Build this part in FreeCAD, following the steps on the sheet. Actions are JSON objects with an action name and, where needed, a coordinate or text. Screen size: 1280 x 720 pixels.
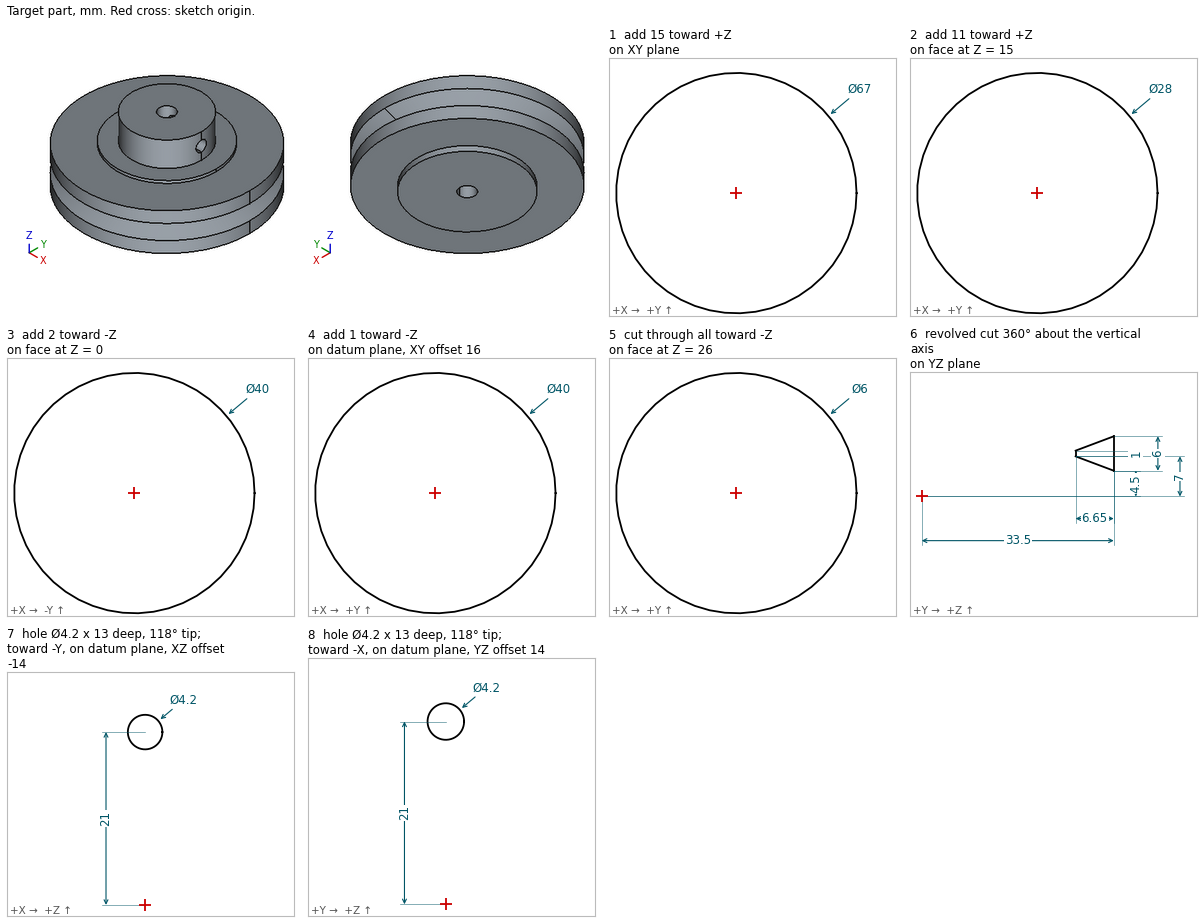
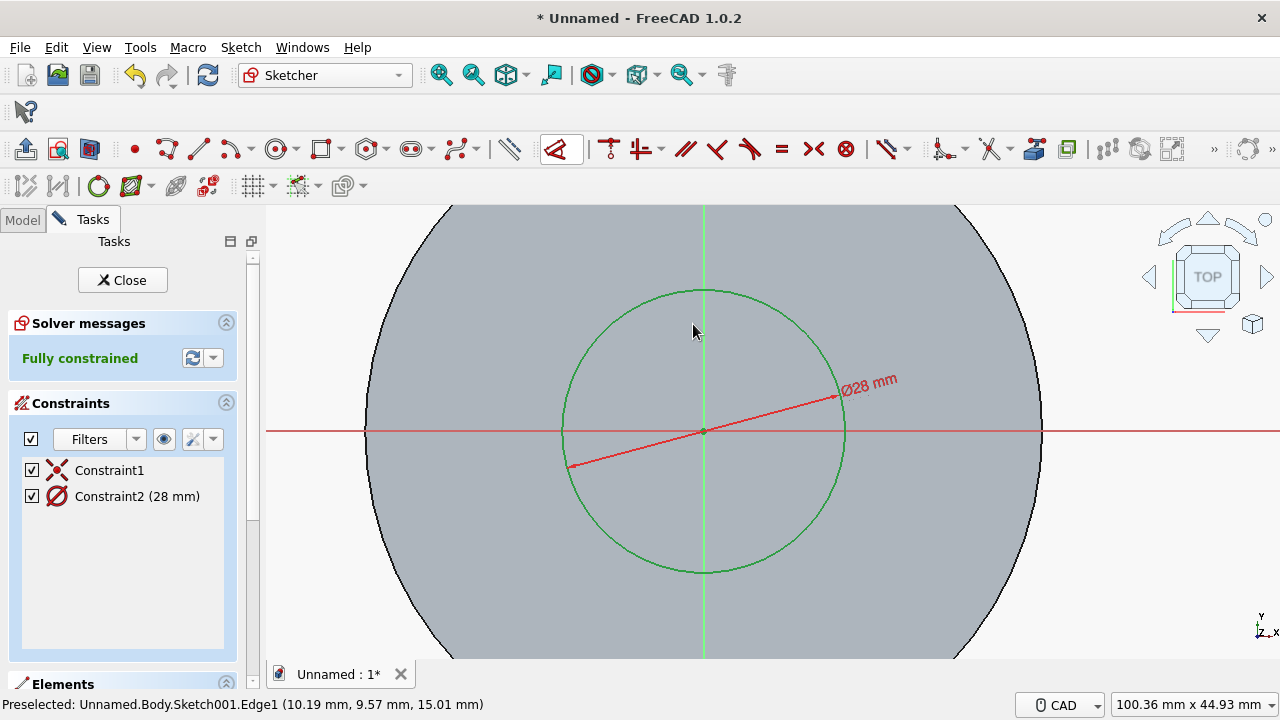
{"action": "left_click", "coordinate": [123, 280]}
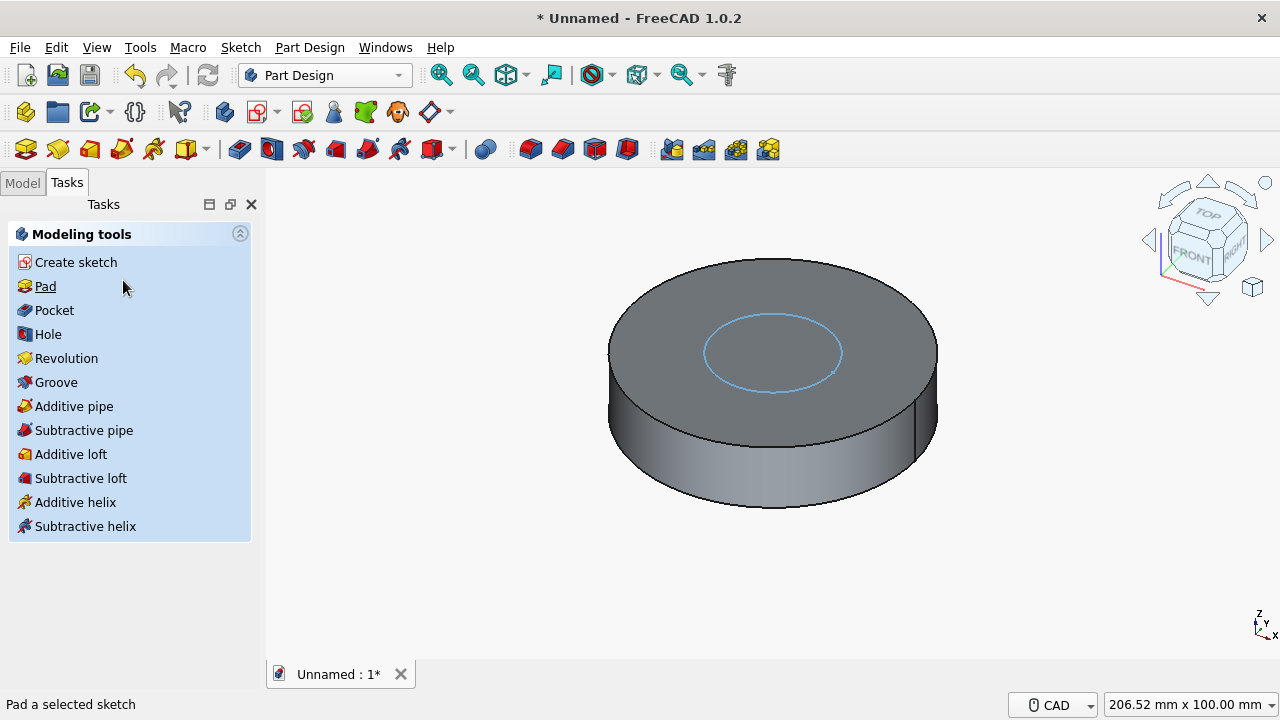
{"action": "left_click", "coordinate": [26, 150]}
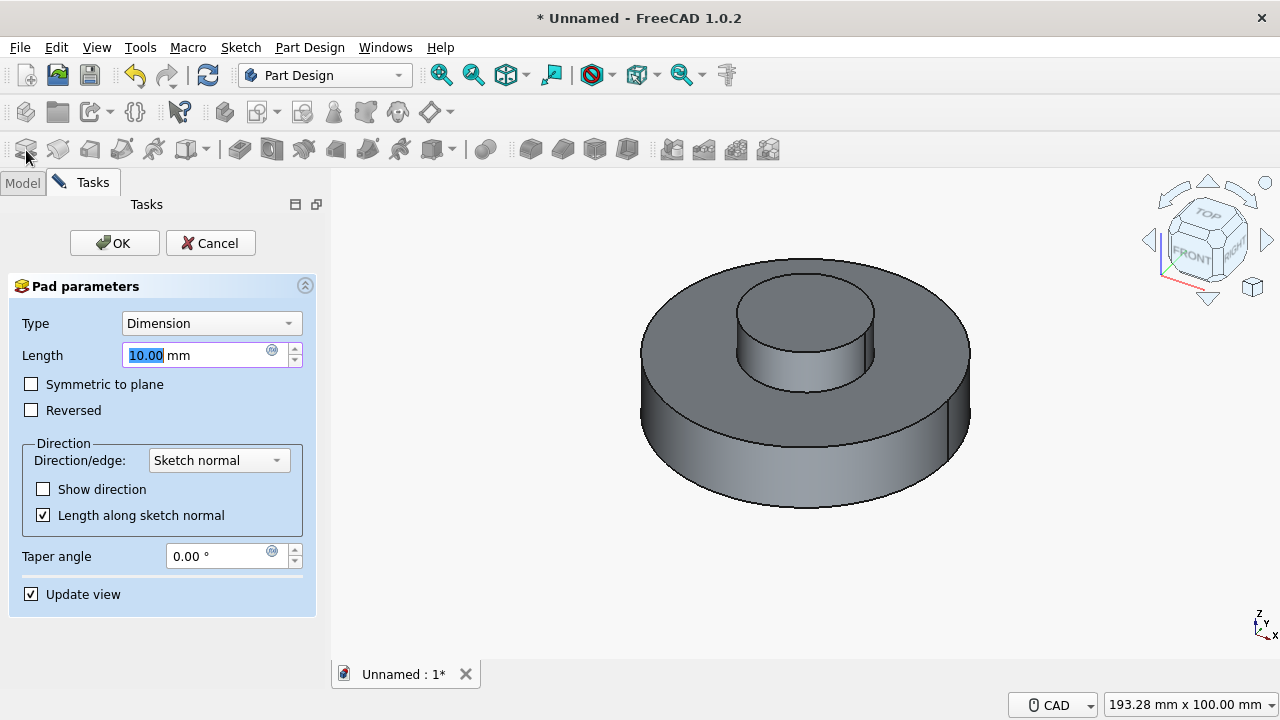
{"action": "type", "text": "11"}
{"action": "key", "text": "Tab"}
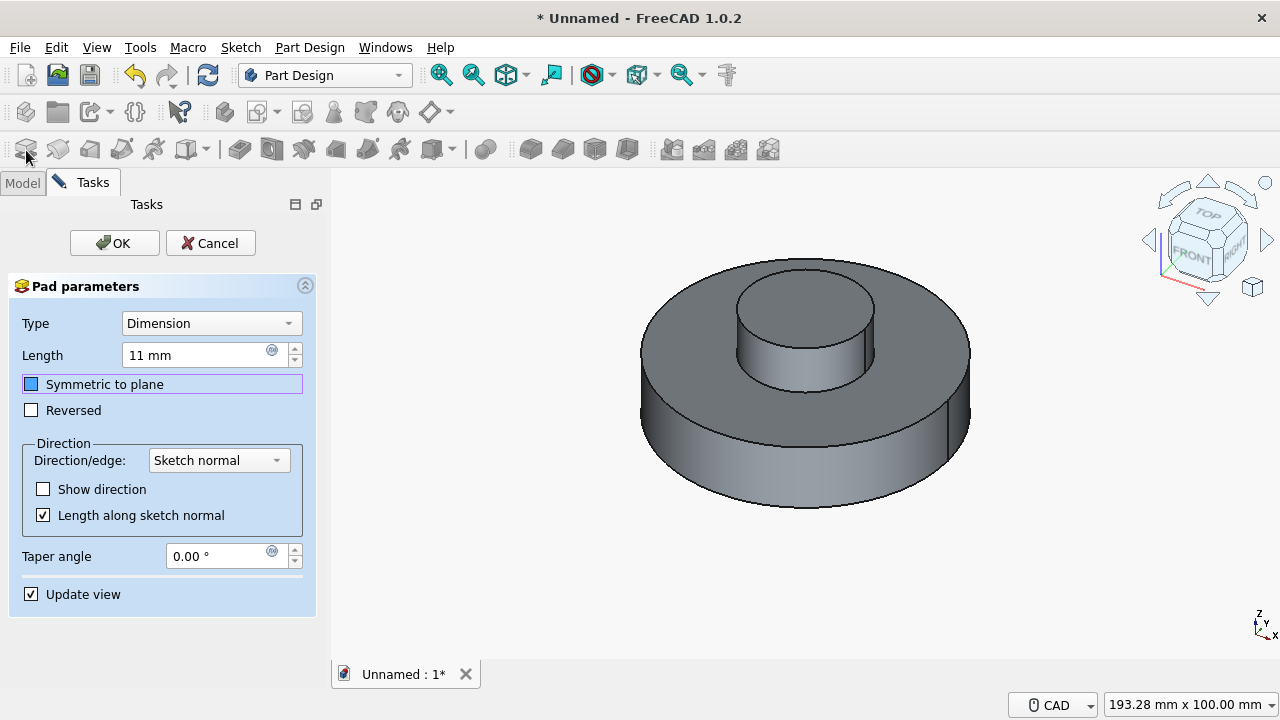
{"action": "left_click", "coordinate": [115, 243]}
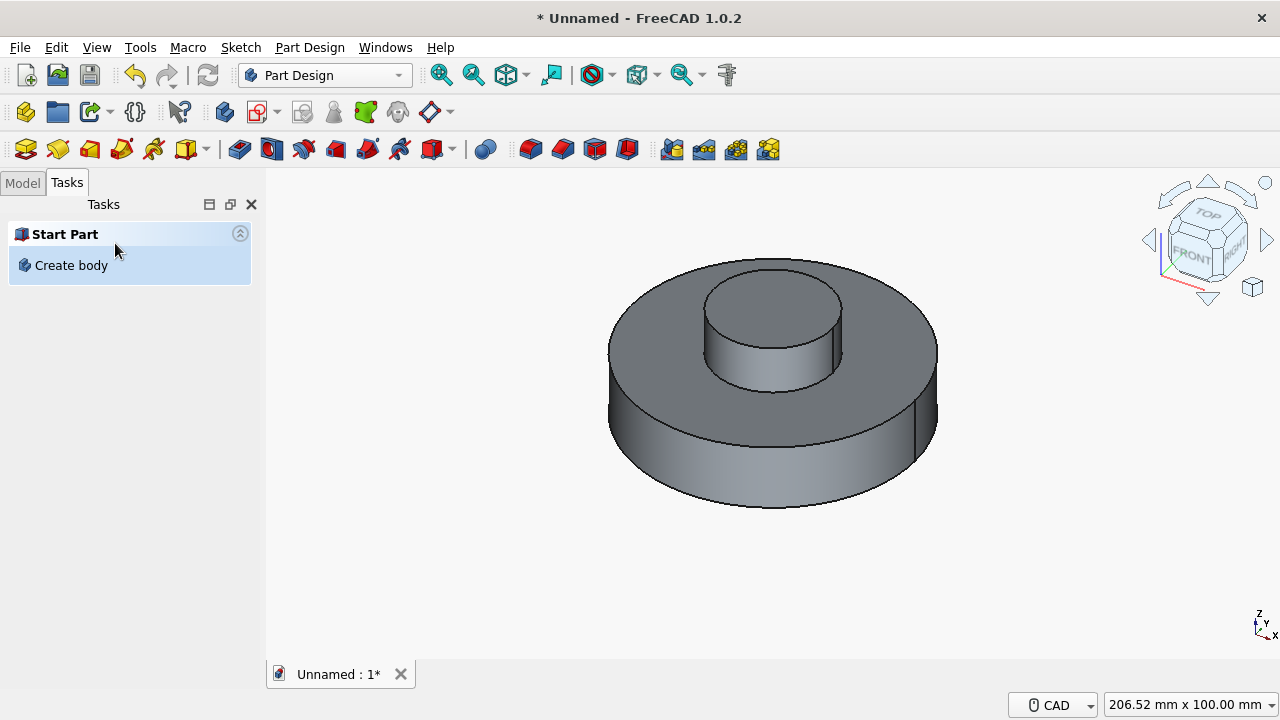
{"action": "key", "text": "5"}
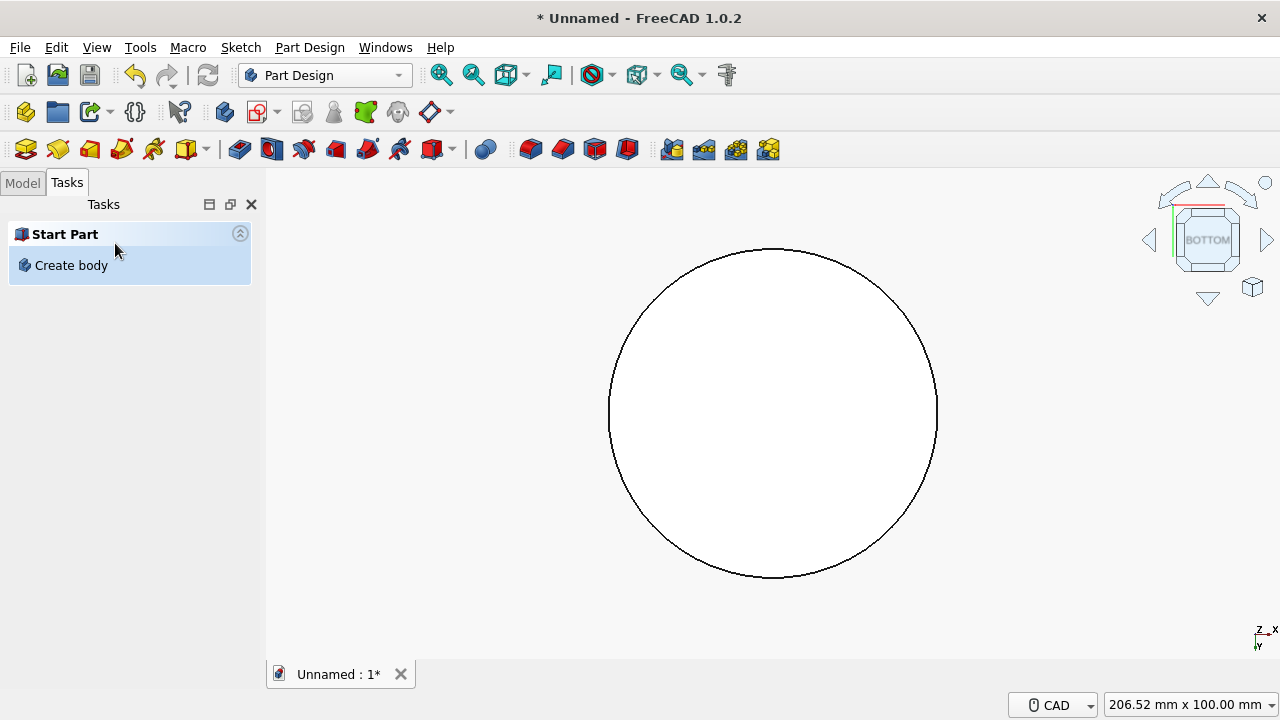
{"action": "left_click", "coordinate": [773, 412]}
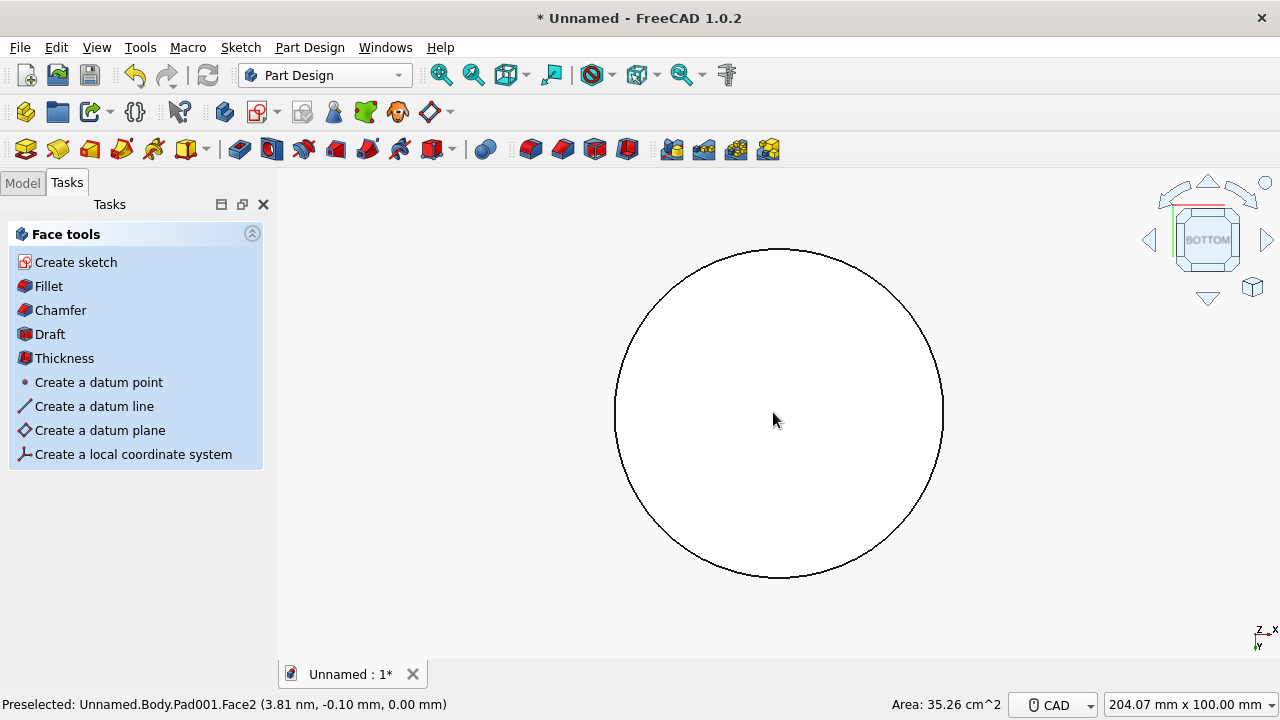
{"action": "left_click", "coordinate": [258, 112]}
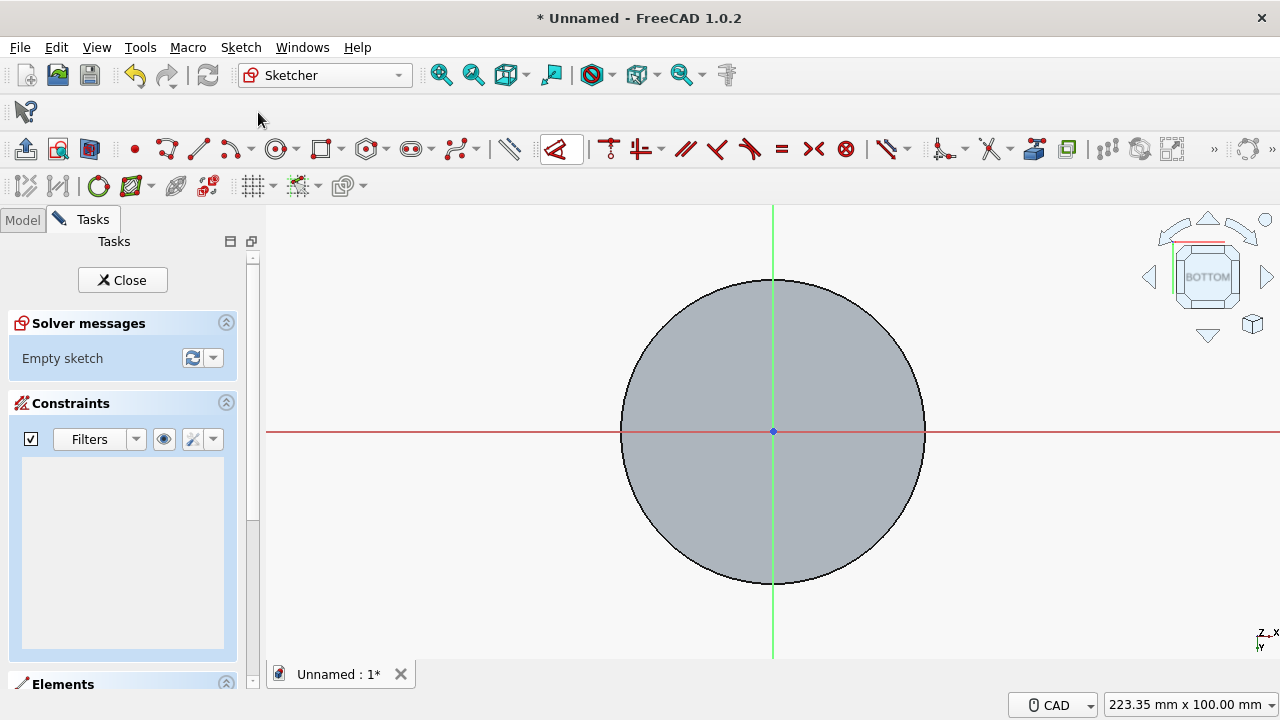
{"action": "scroll", "coordinate": [912, 432], "scroll_direction": "up", "scroll_amount": 2}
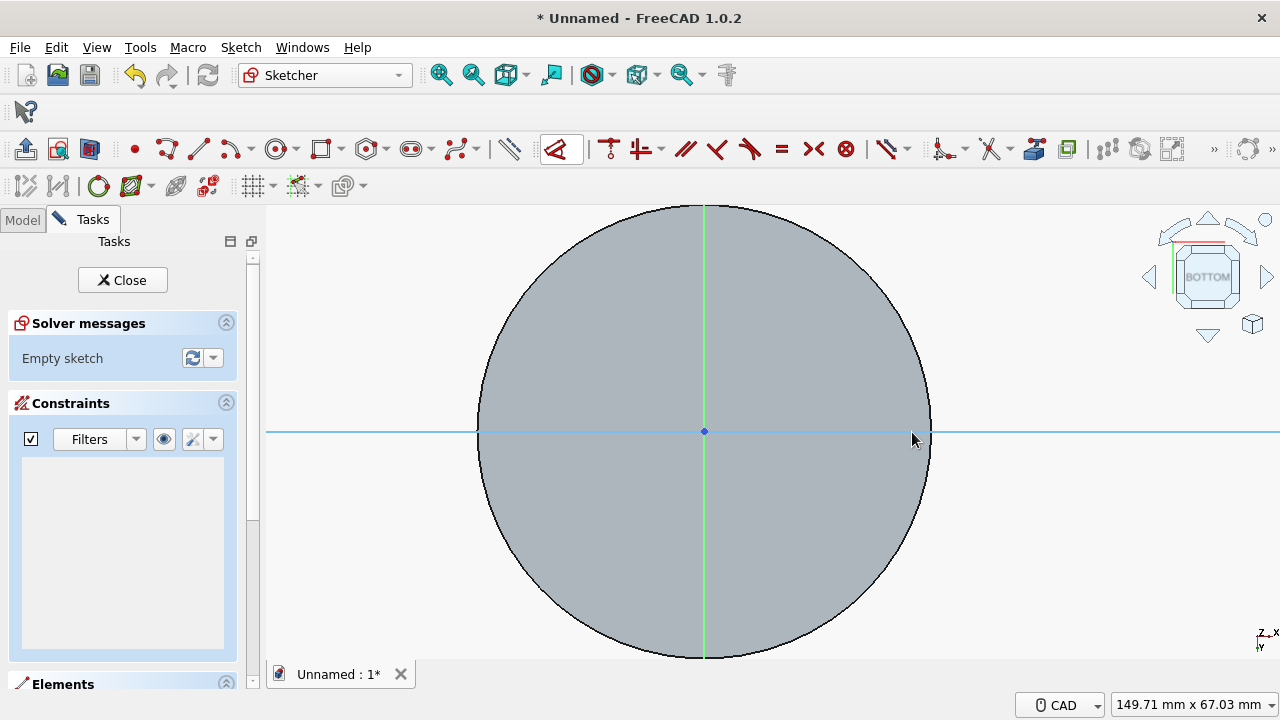
{"action": "left_click", "coordinate": [276, 150]}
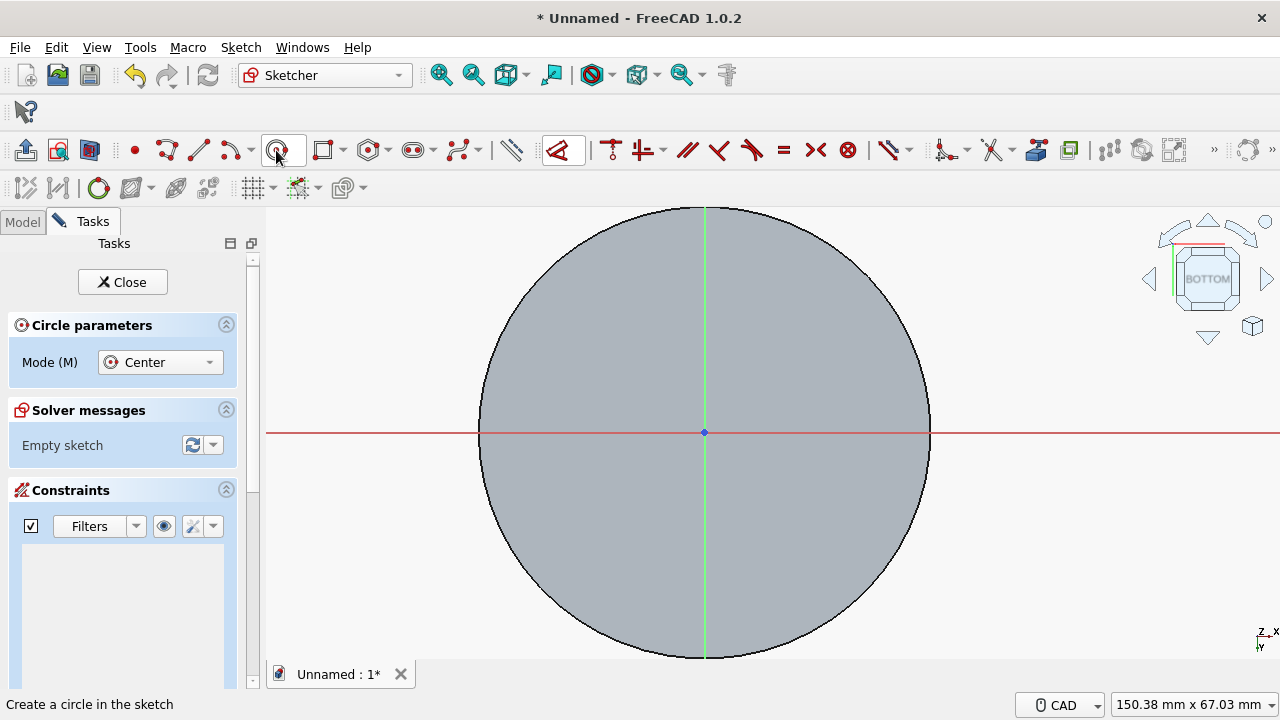
{"action": "left_click", "coordinate": [705, 433]}
{"action": "left_click", "coordinate": [800, 337]}
{"action": "key", "text": "Escape"}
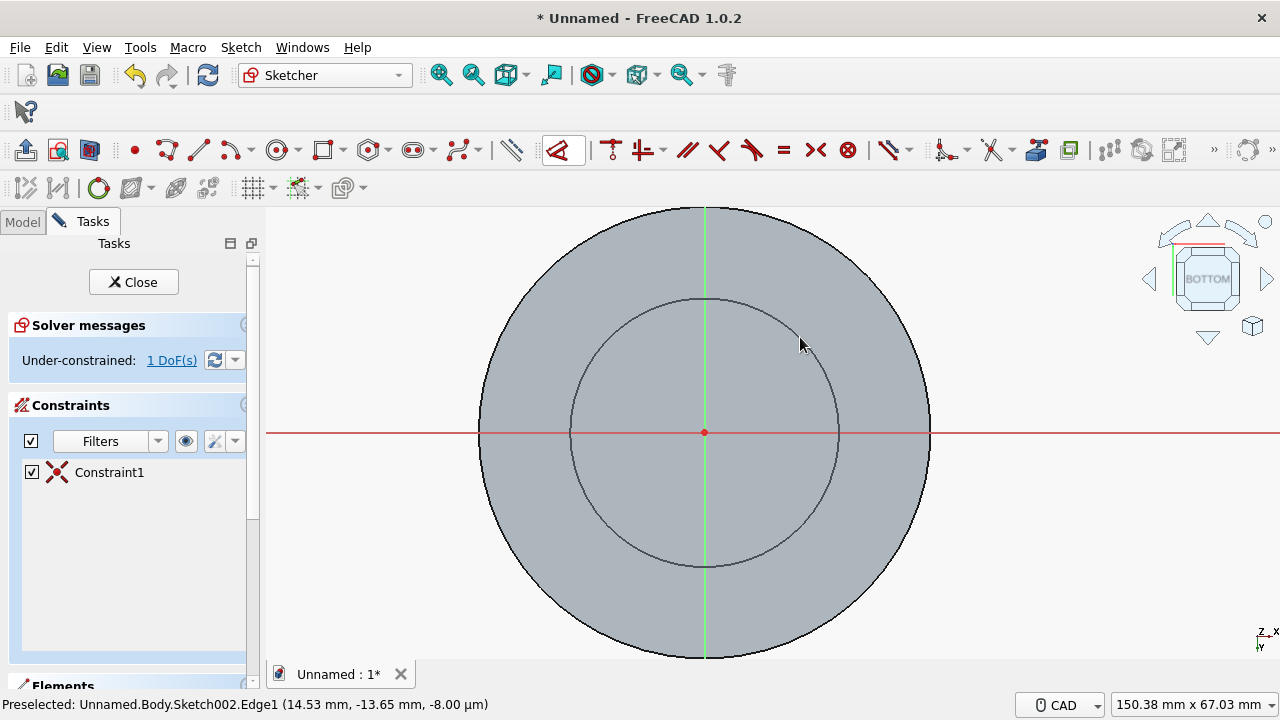
{"action": "left_click", "coordinate": [799, 337]}